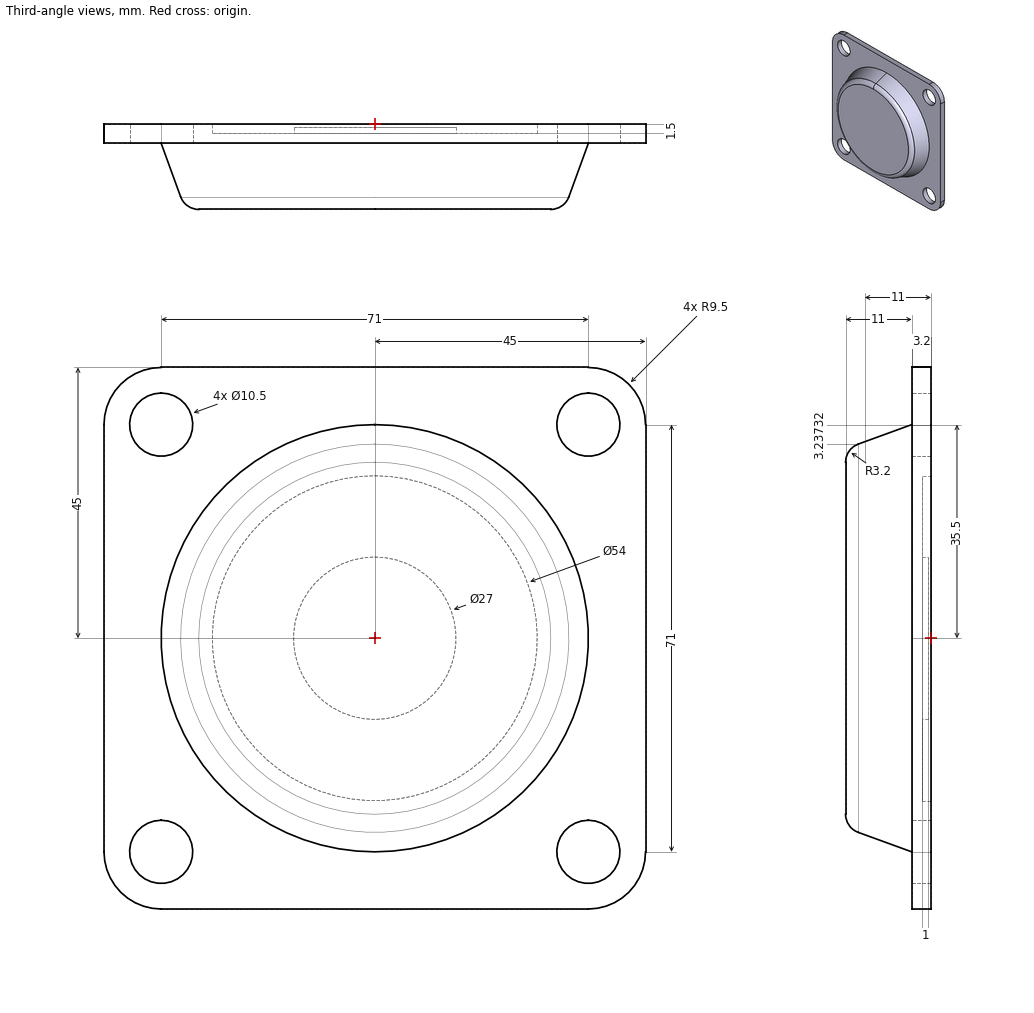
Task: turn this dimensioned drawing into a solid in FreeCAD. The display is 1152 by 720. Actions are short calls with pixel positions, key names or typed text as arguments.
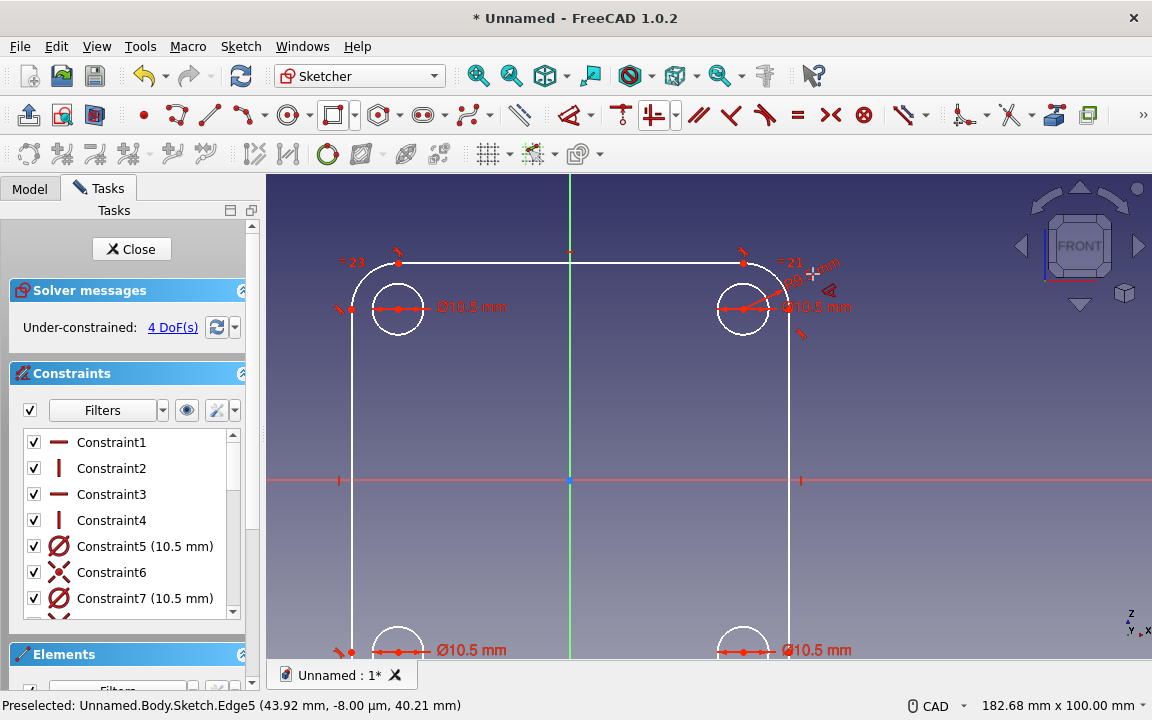
click(502, 263)
click(491, 229)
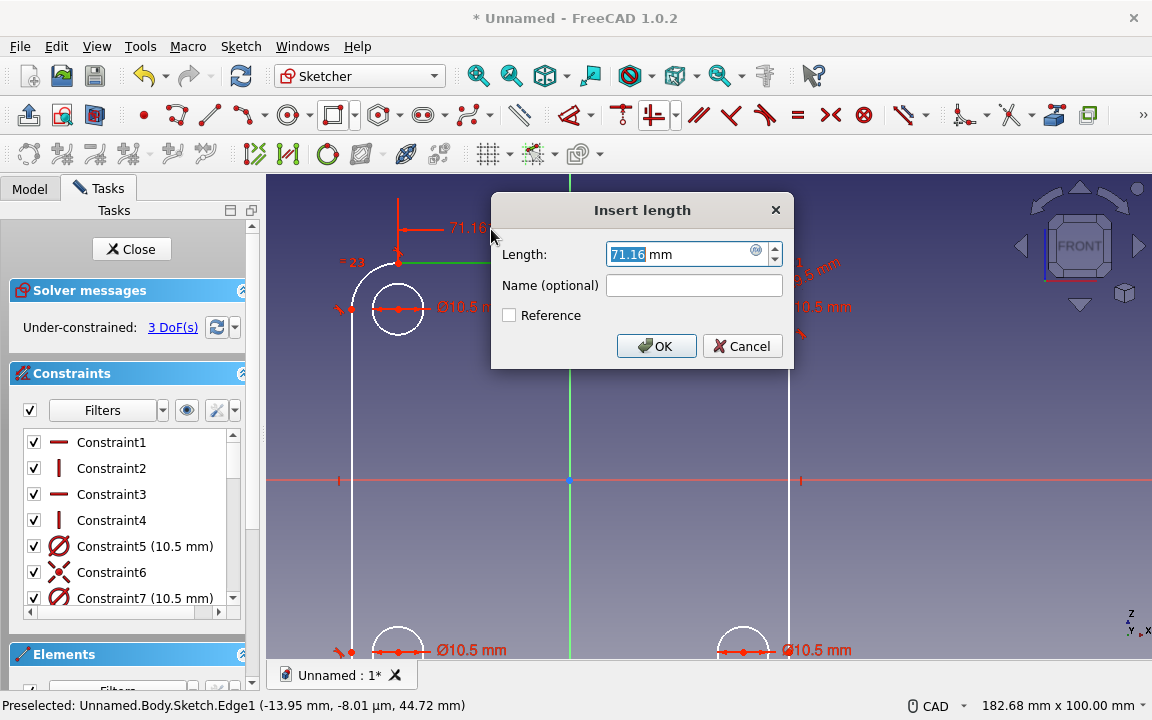
text(71)
key(Return)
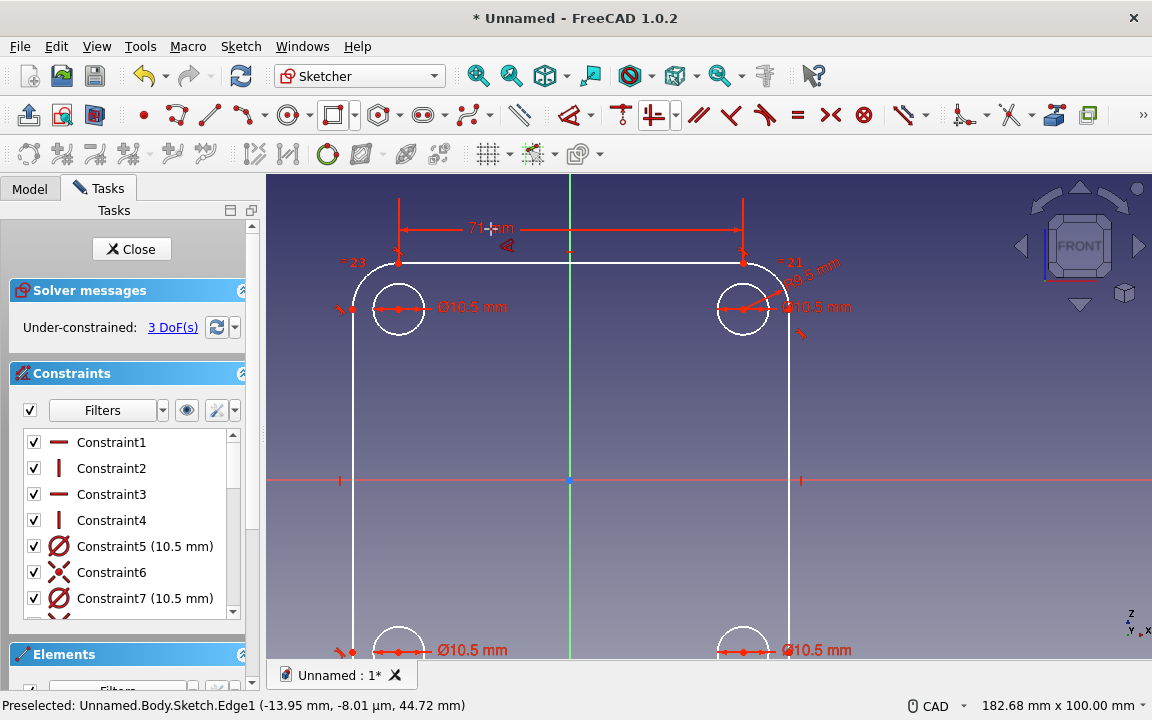
click(789, 412)
click(823, 396)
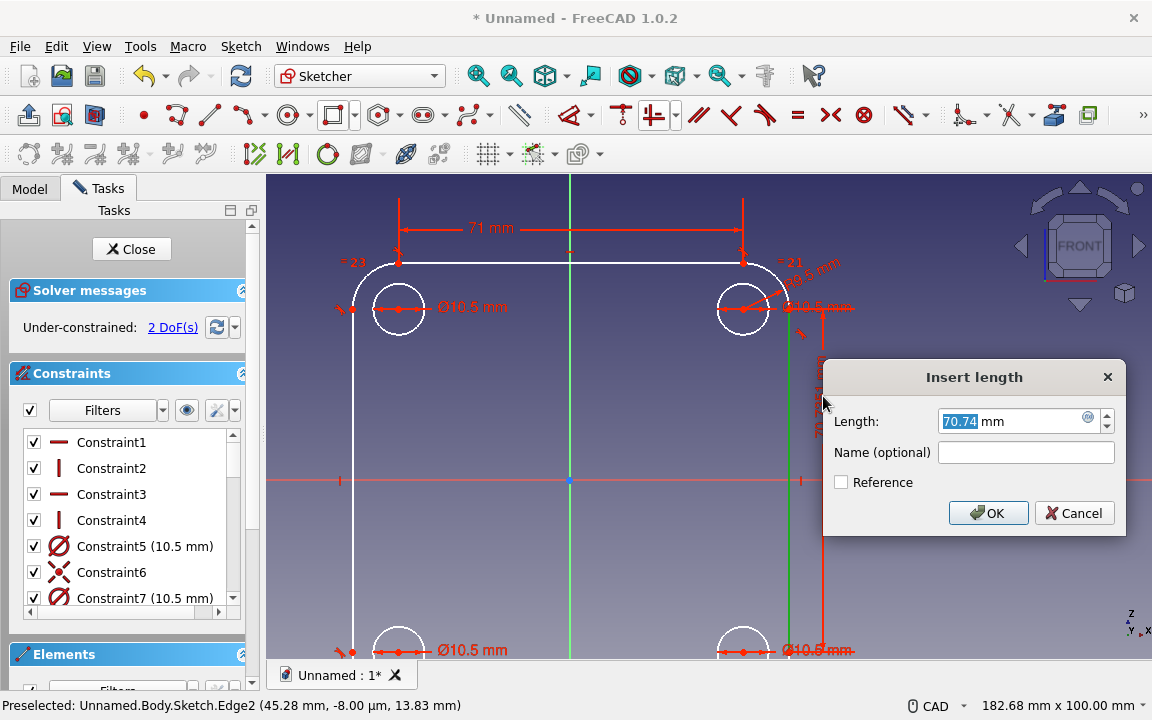
text(71)
key(Return)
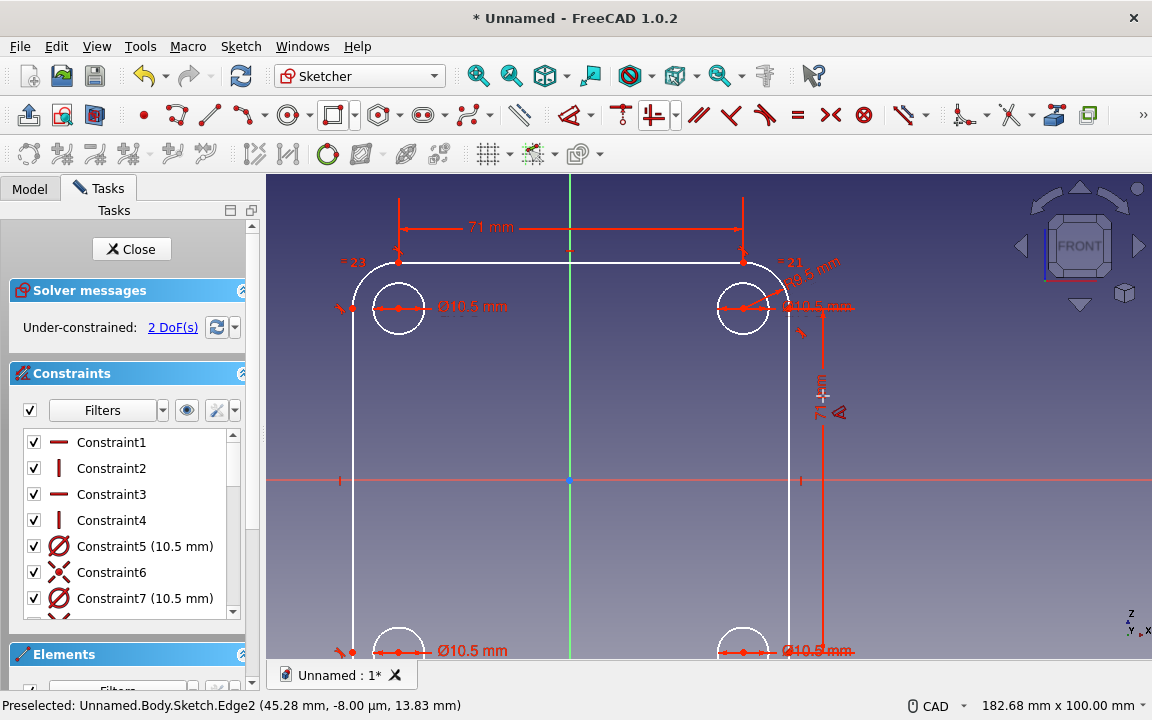
click(399, 263)
click(604, 371)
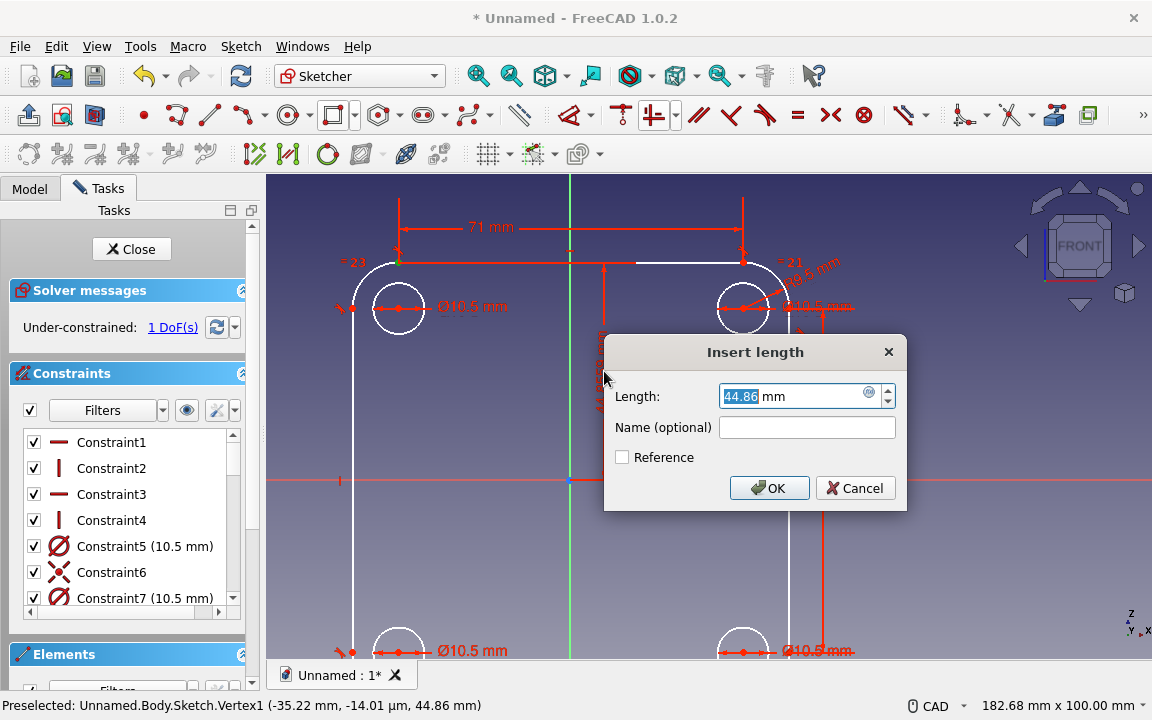
text(45)
key(Return)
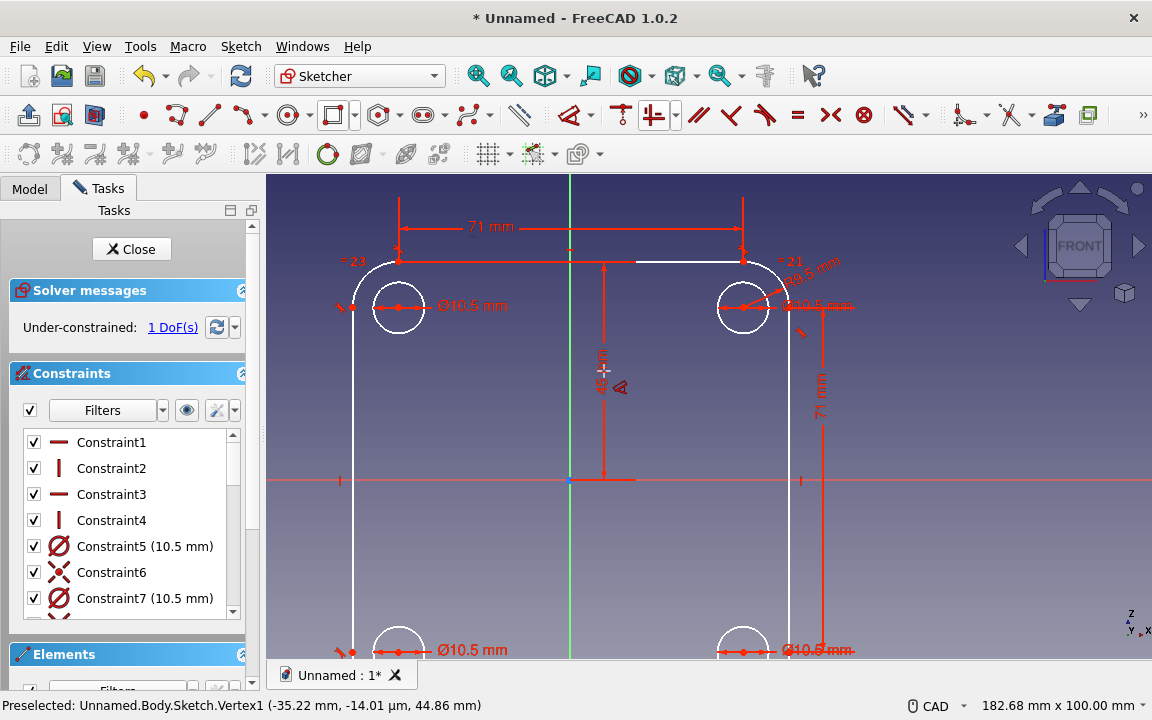
click(789, 308)
click(679, 514)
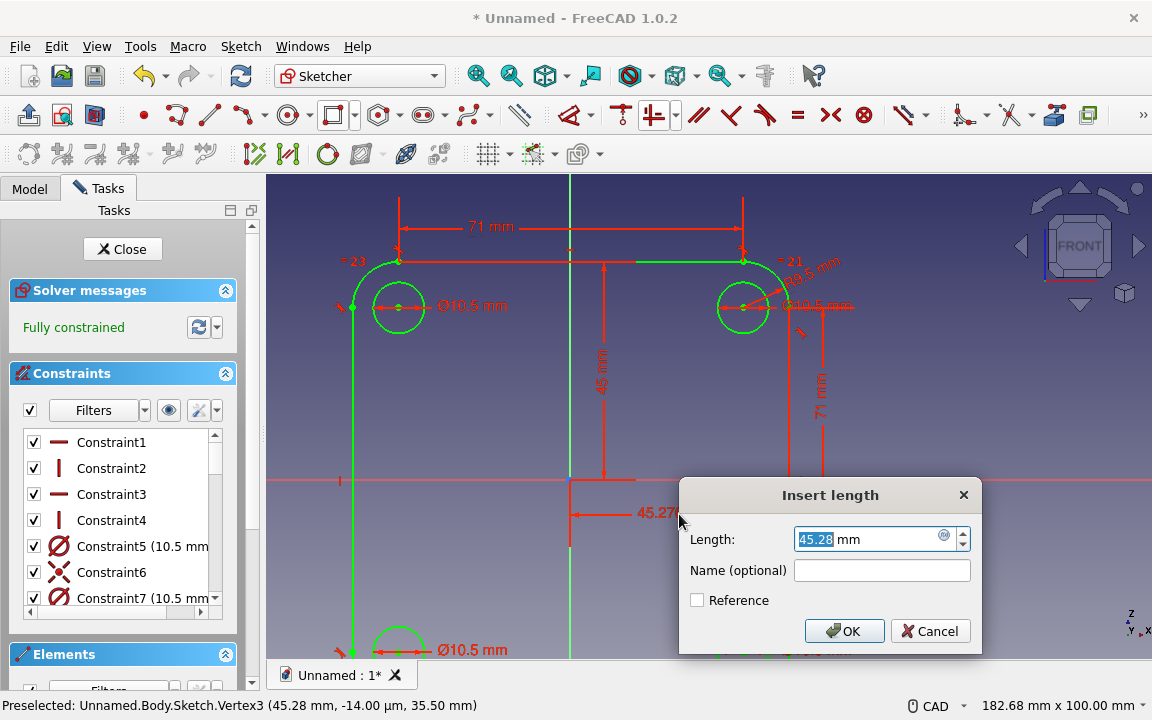
text(45)
key(Return)
key(Escape)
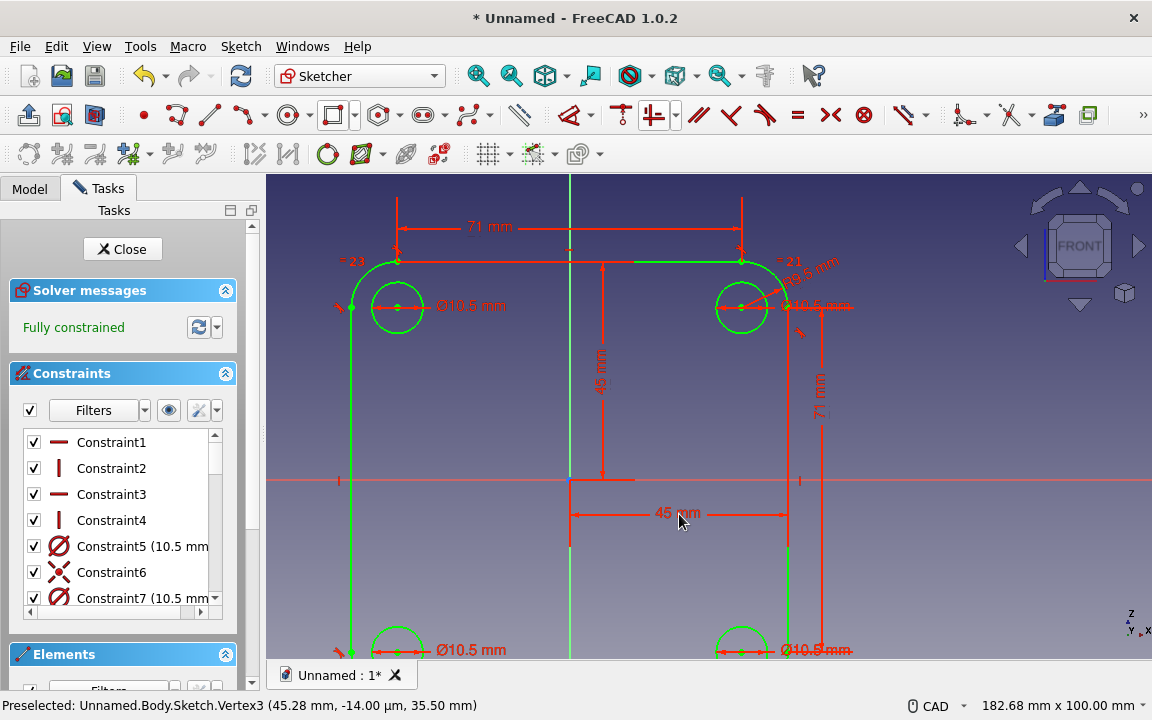
click(123, 249)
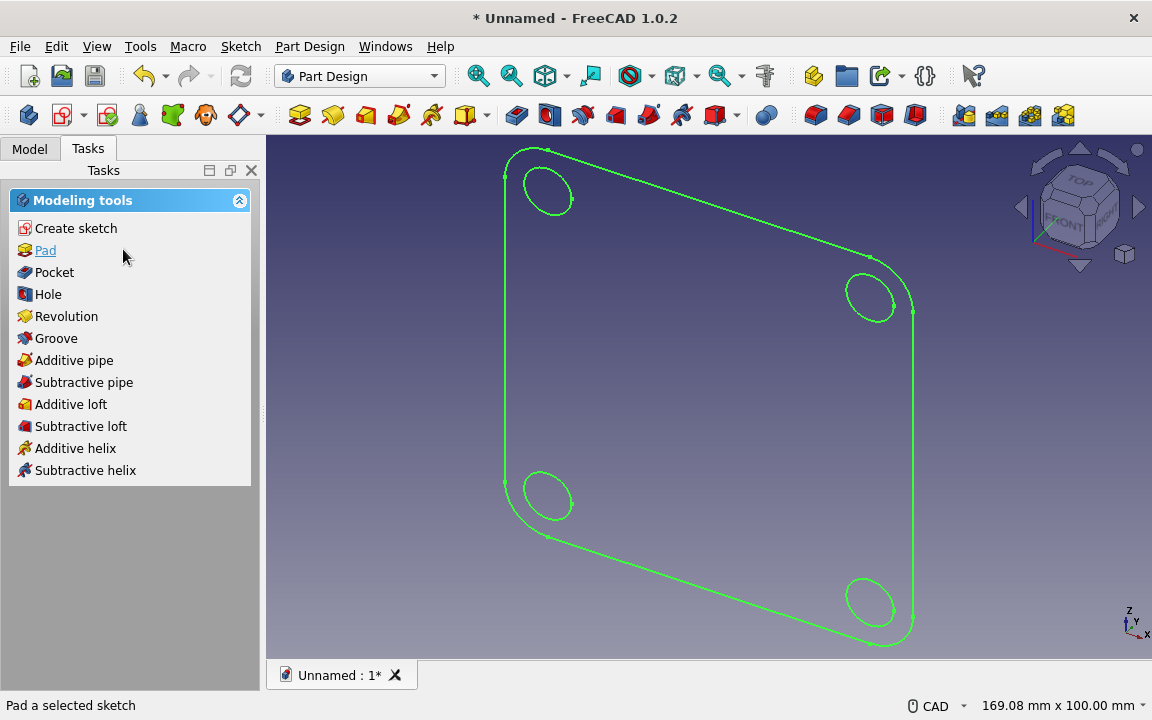
click(300, 116)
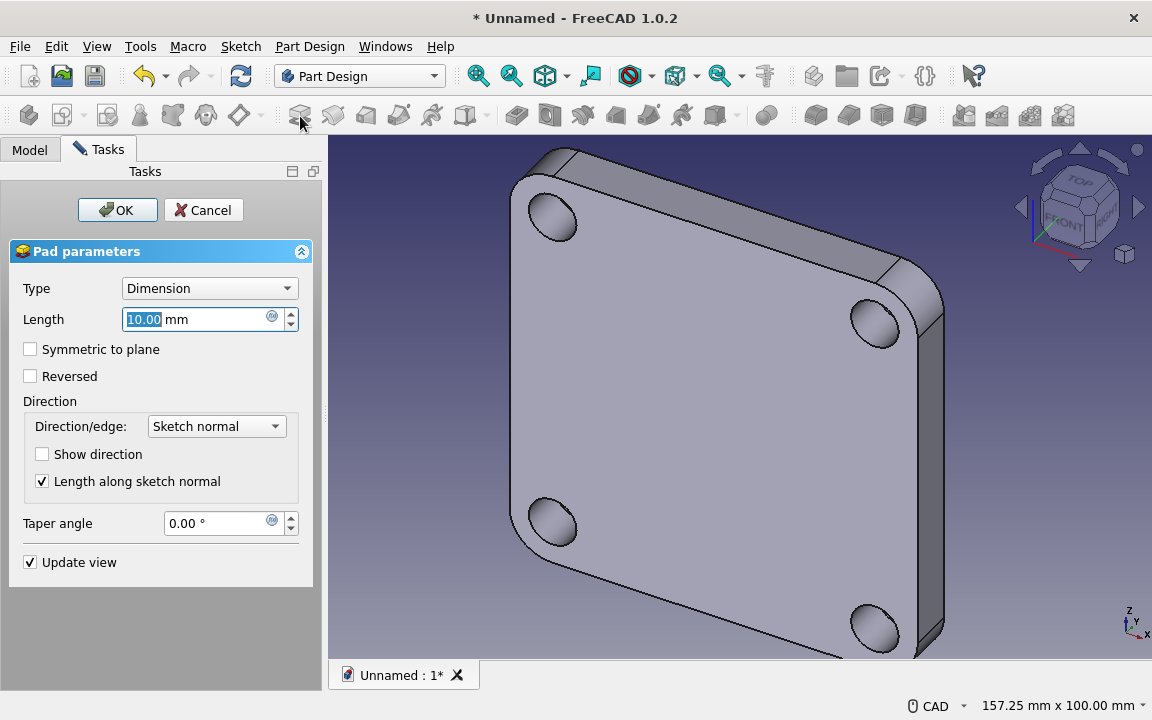
text(3.2)
key(Tab)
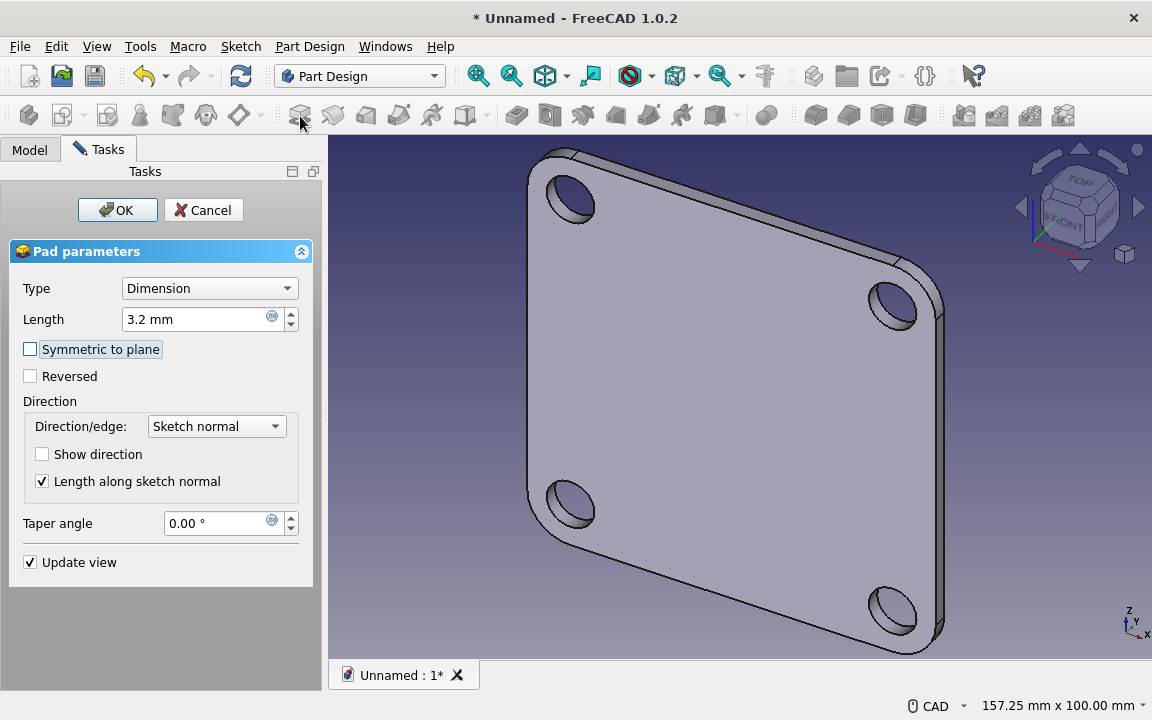
click(118, 210)